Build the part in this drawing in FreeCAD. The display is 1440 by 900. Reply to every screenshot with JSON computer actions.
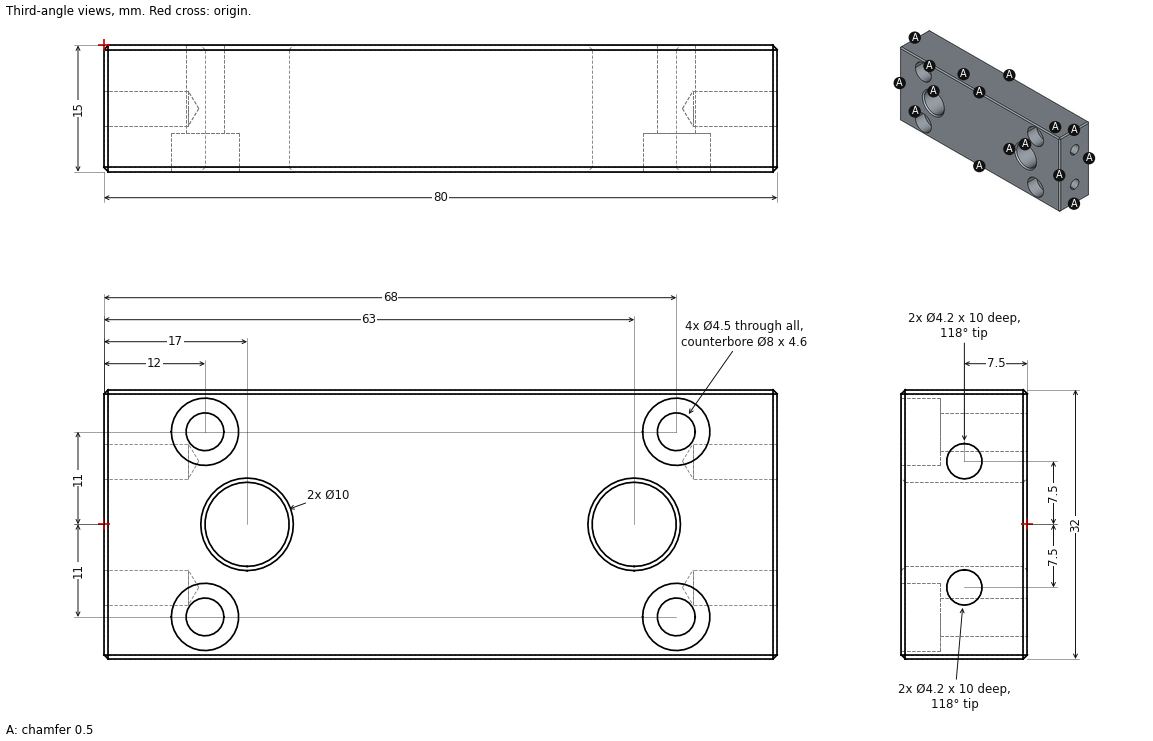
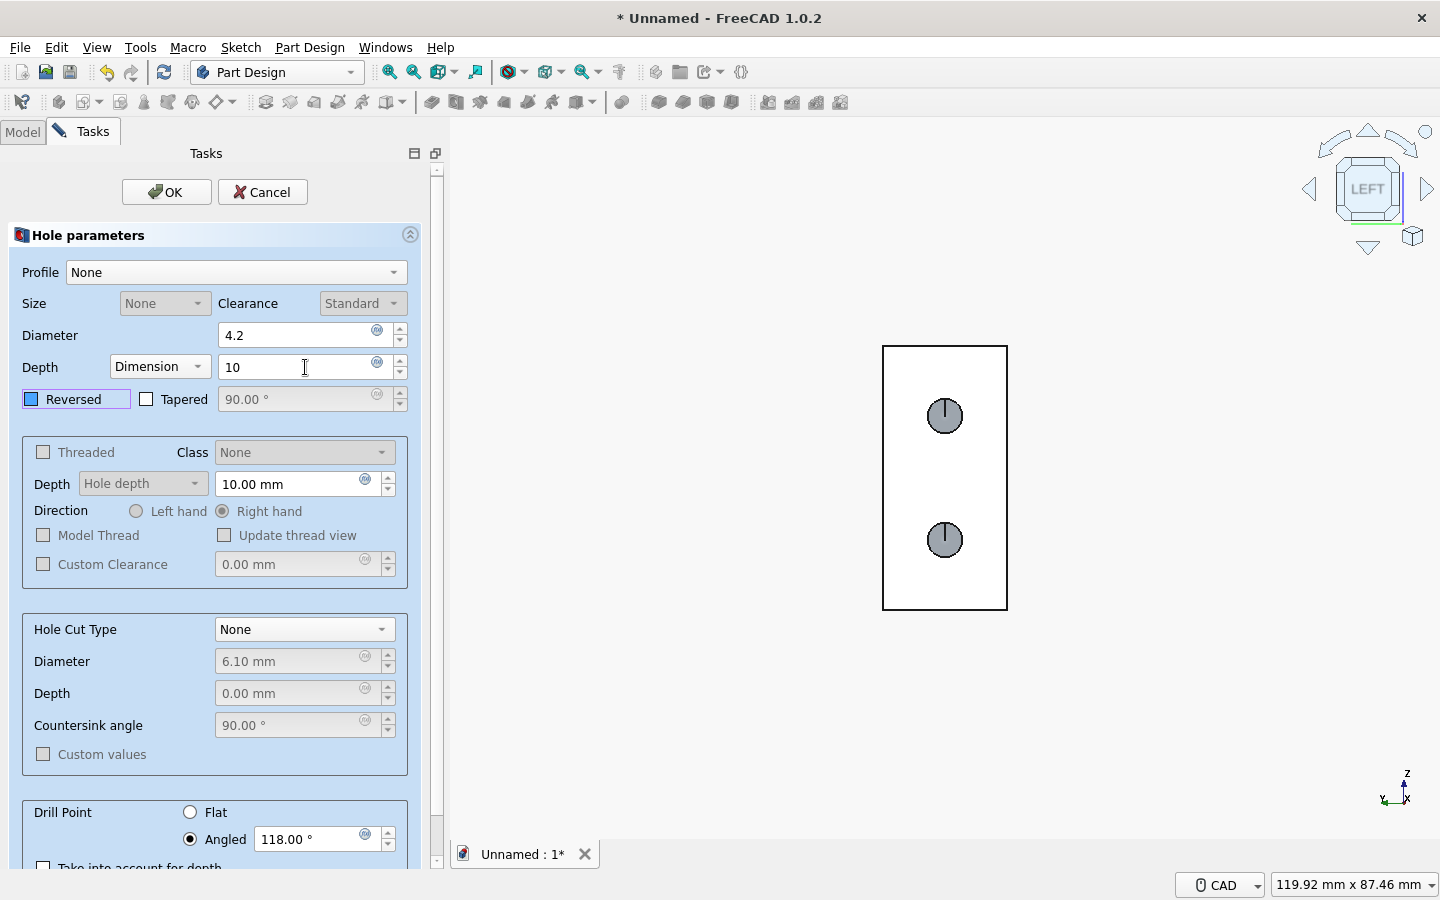
{"action": "left_click", "coordinate": [167, 192]}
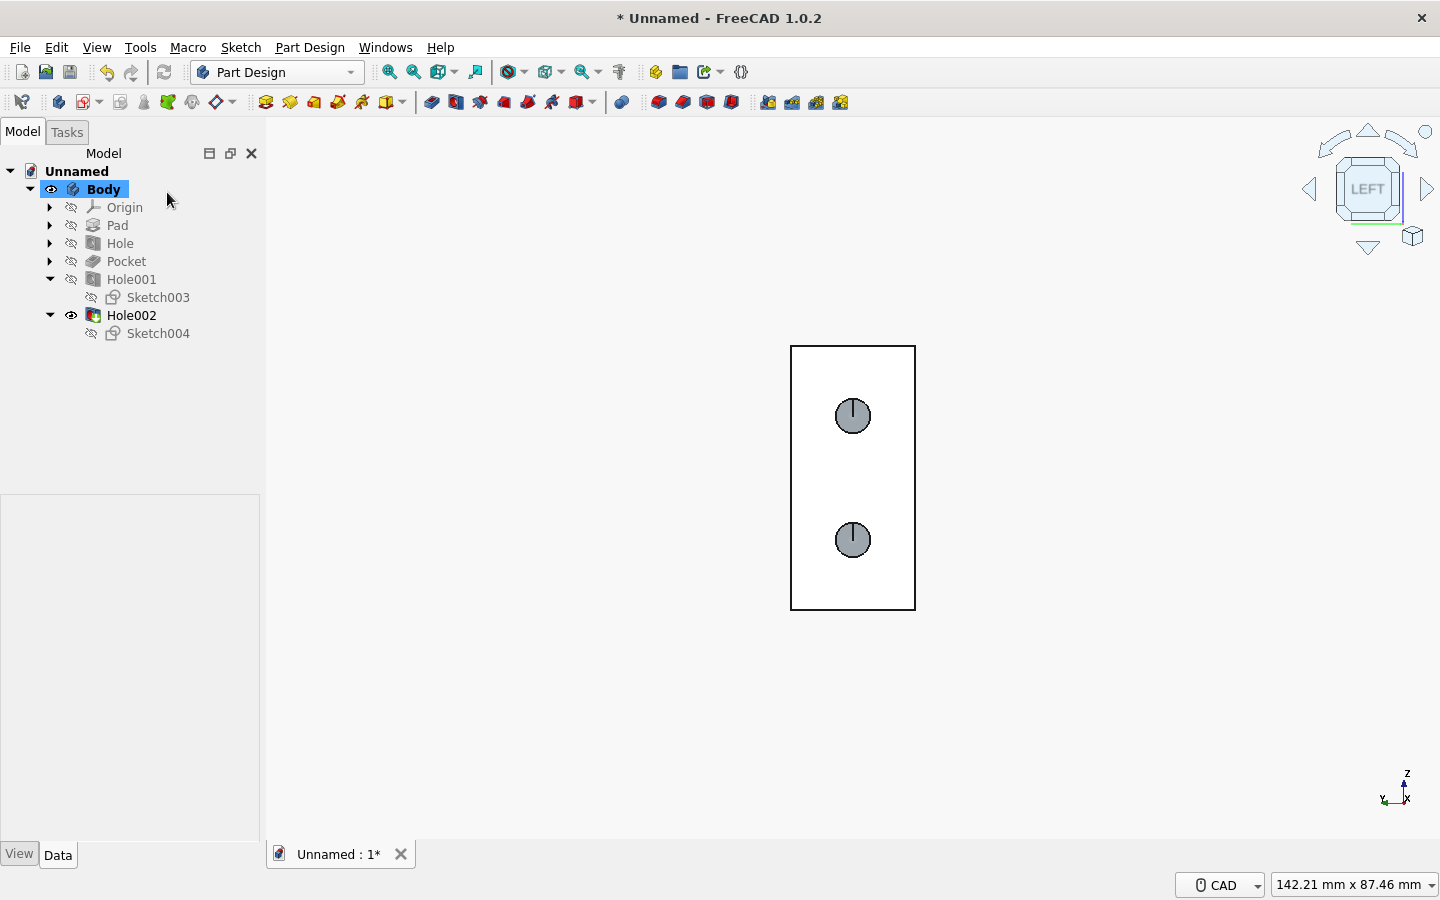
{"action": "left_click", "coordinate": [390, 72]}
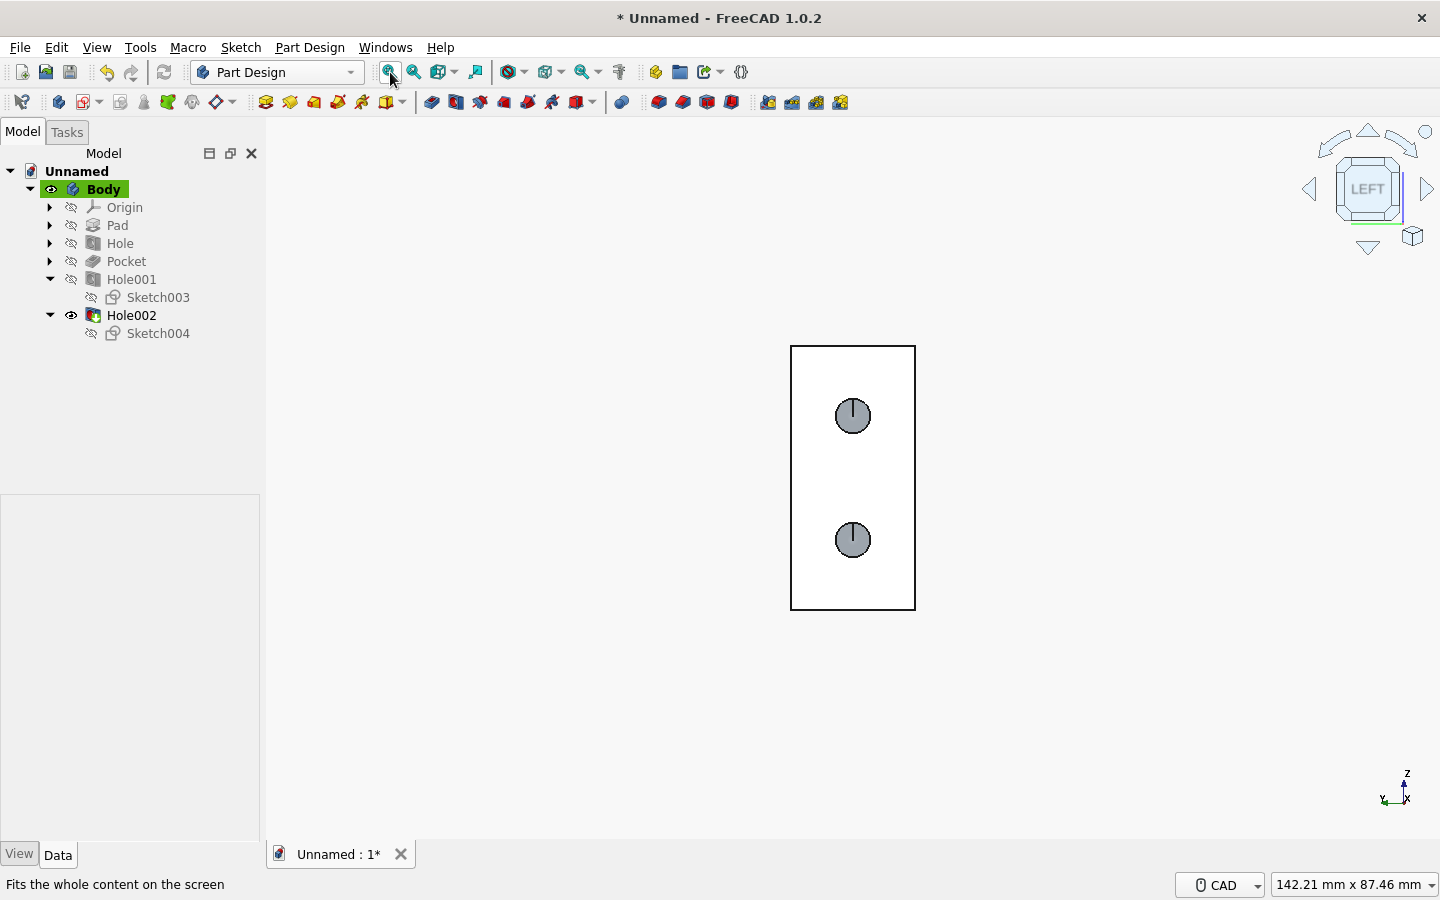
{"action": "left_click", "coordinate": [915, 477]}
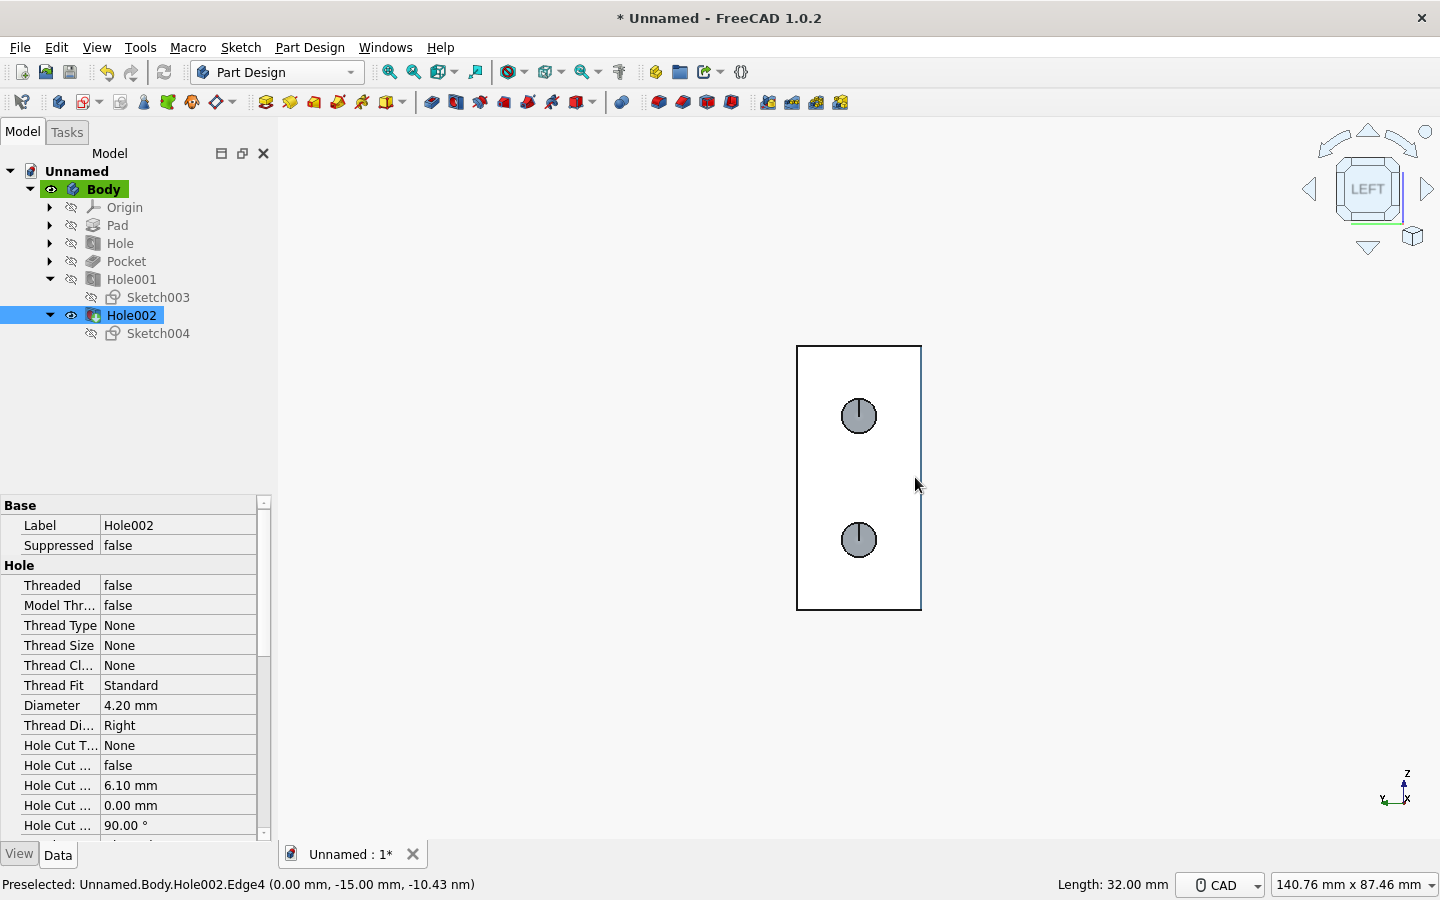
{"action": "left_click", "coordinate": [797, 477], "text": "ctrl"}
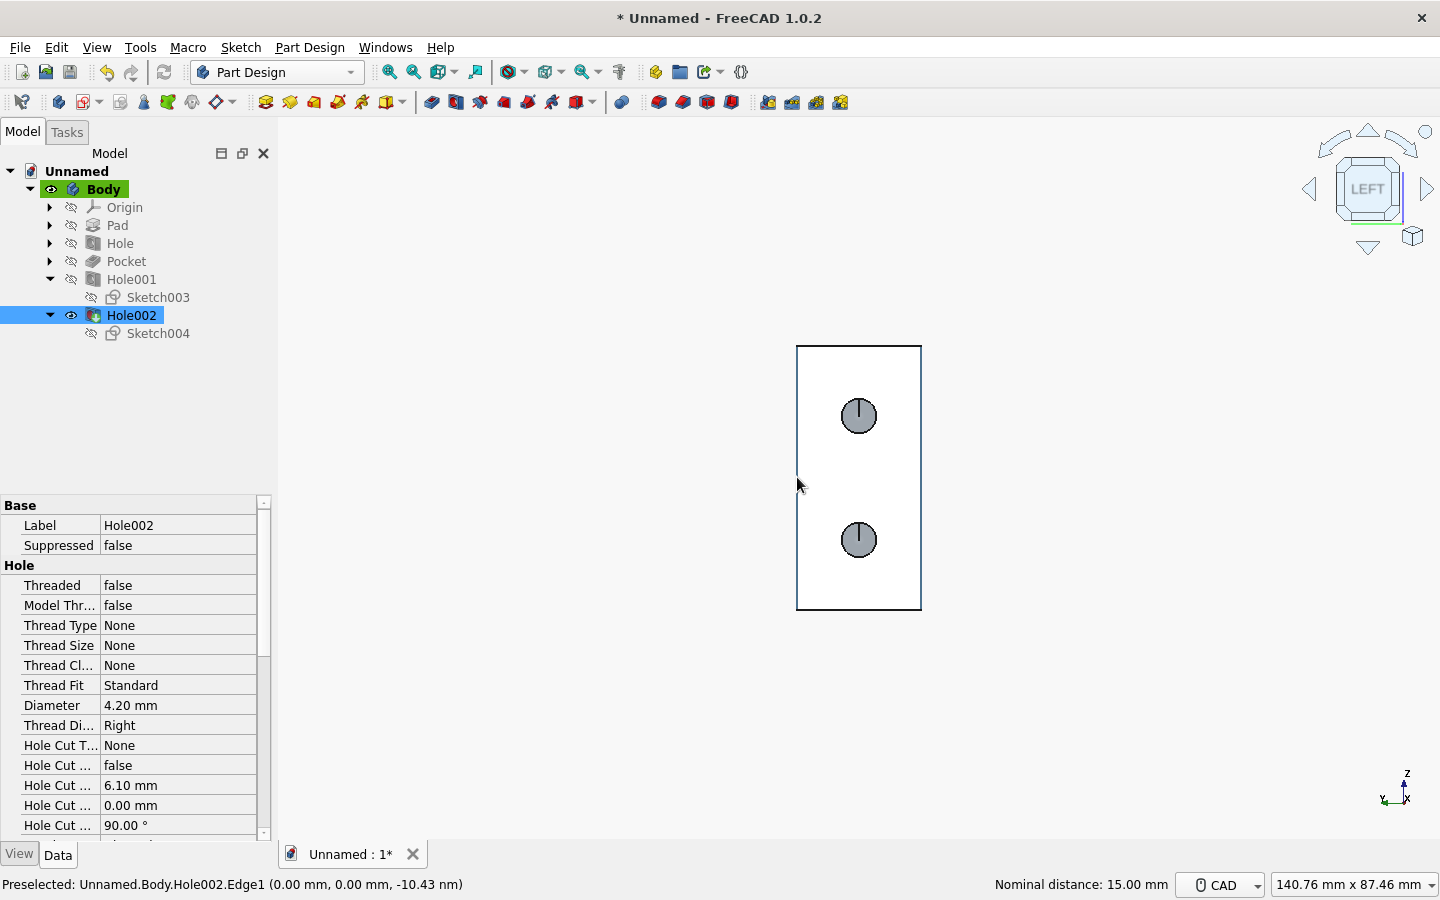
{"action": "key", "text": "0"}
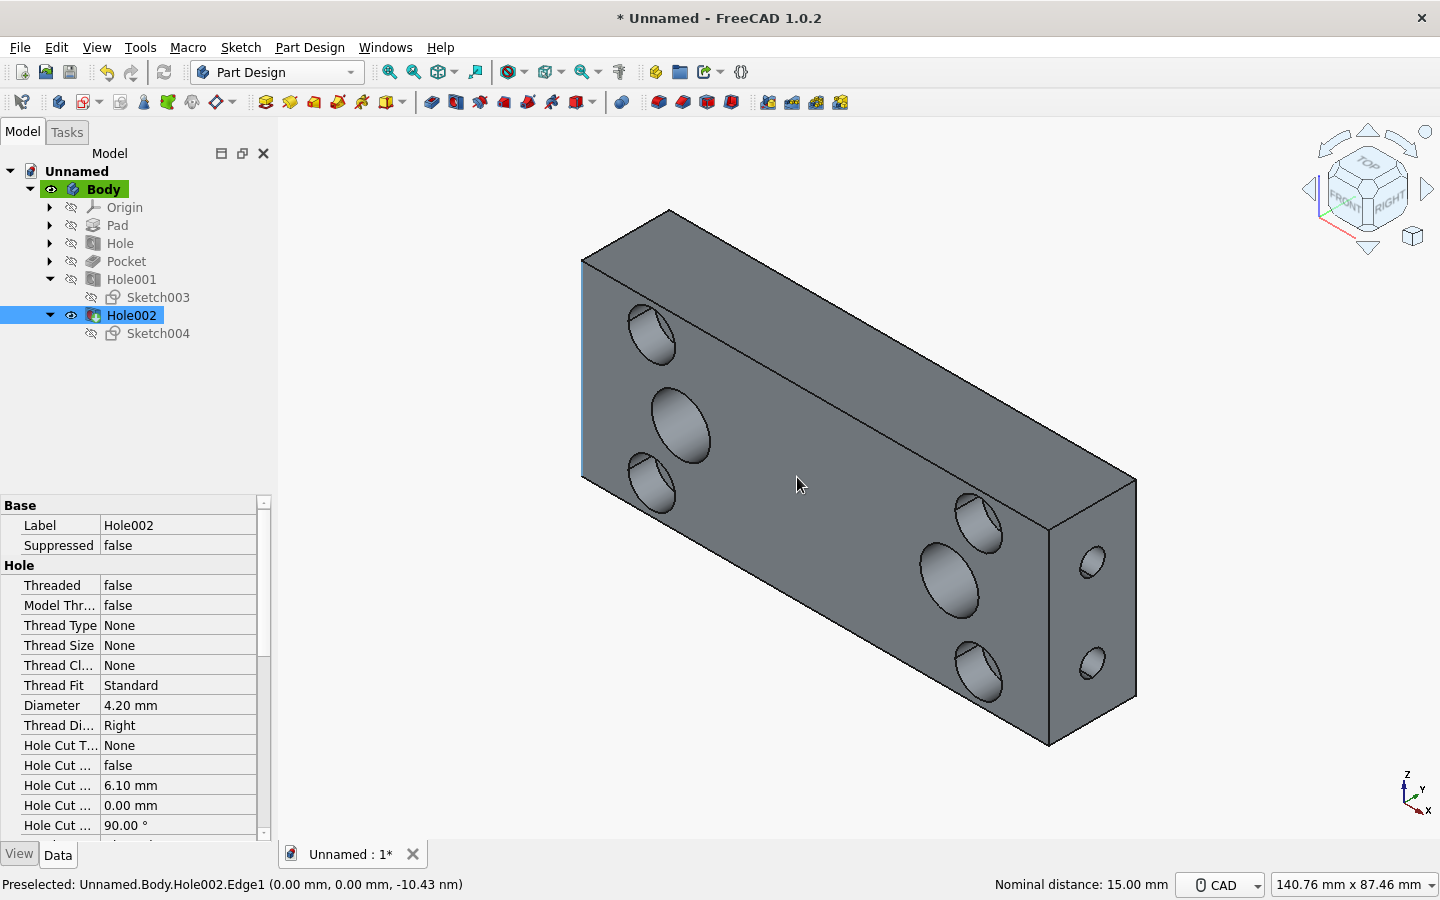
{"action": "left_click", "coordinate": [992, 446], "text": "ctrl"}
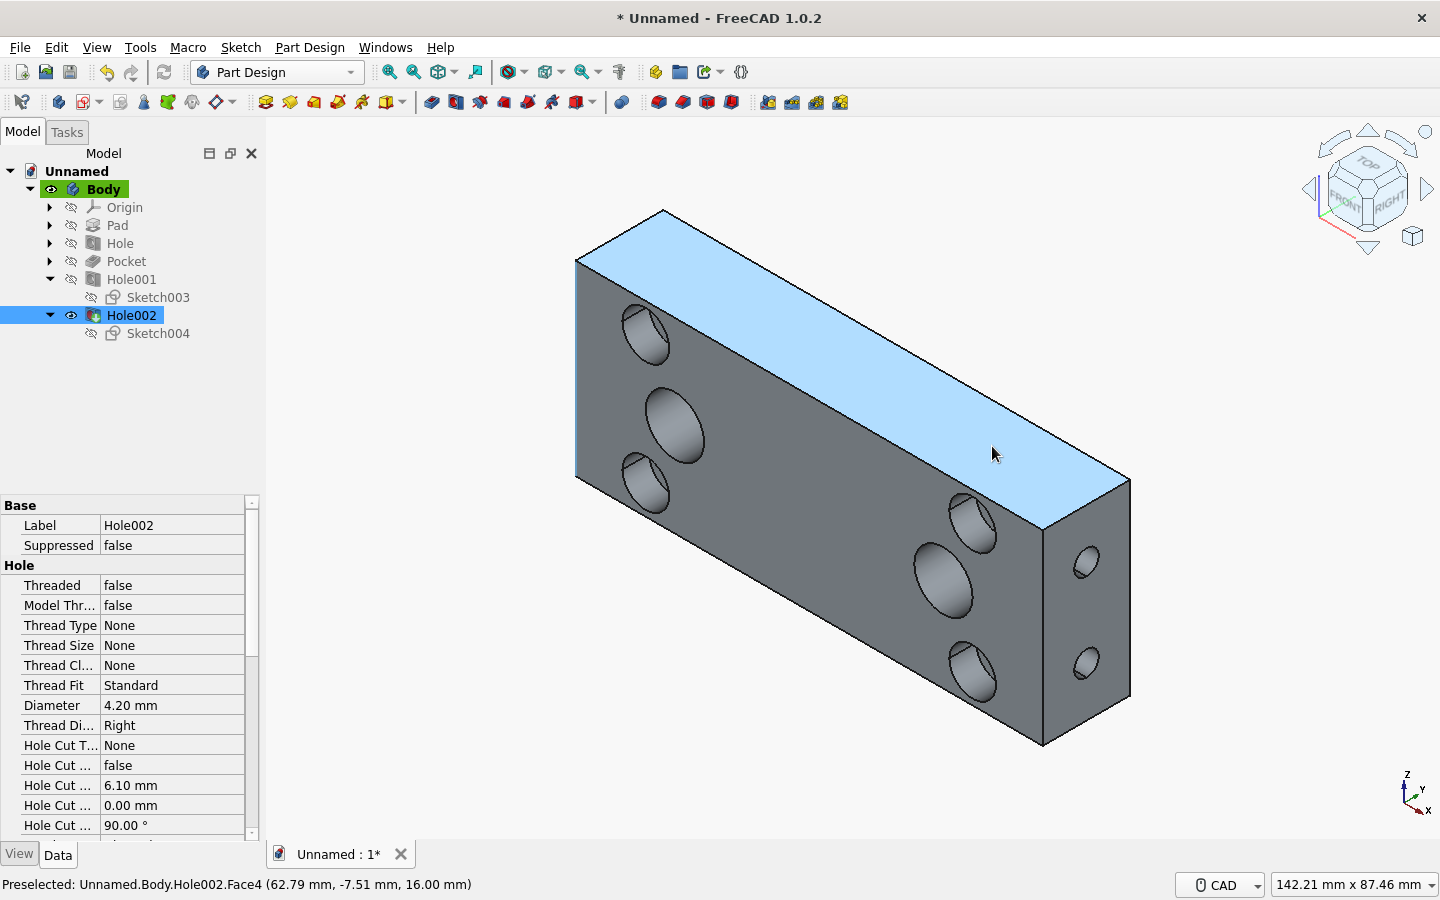
{"action": "left_click", "coordinate": [646, 408], "text": "ctrl"}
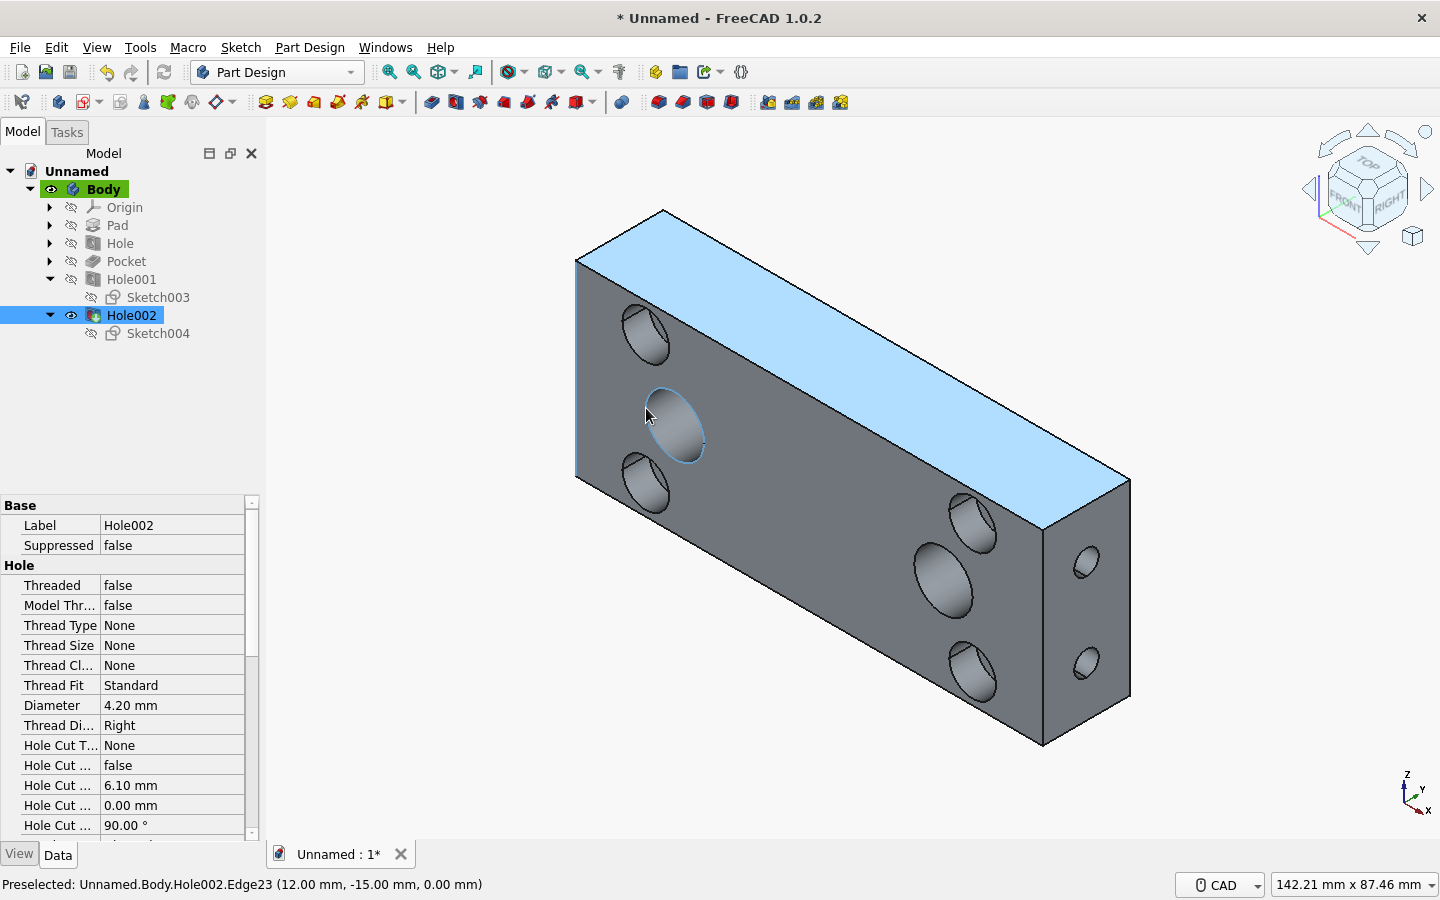
{"action": "left_click", "coordinate": [914, 563], "text": "ctrl"}